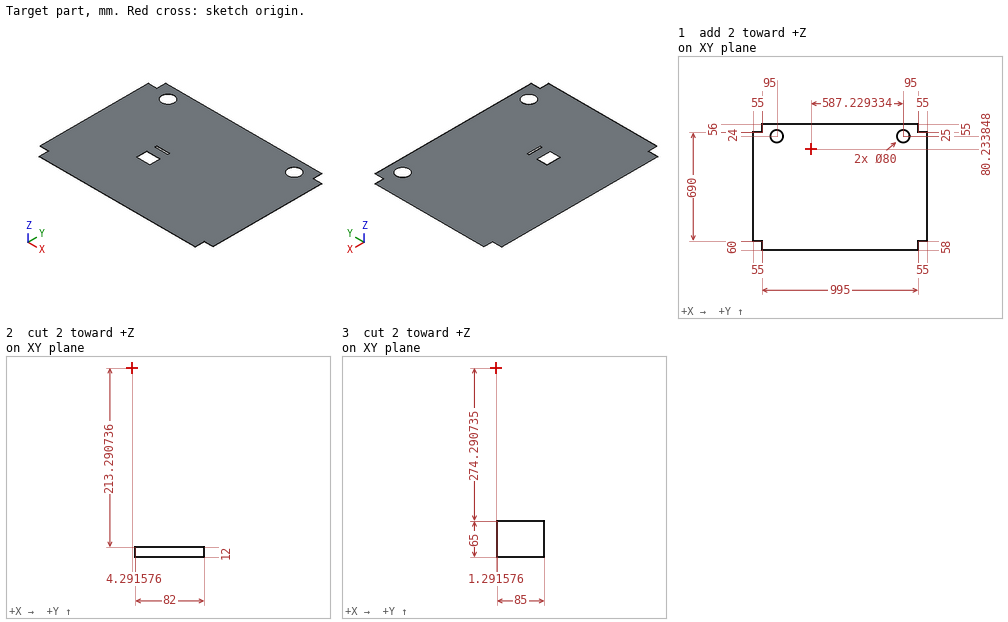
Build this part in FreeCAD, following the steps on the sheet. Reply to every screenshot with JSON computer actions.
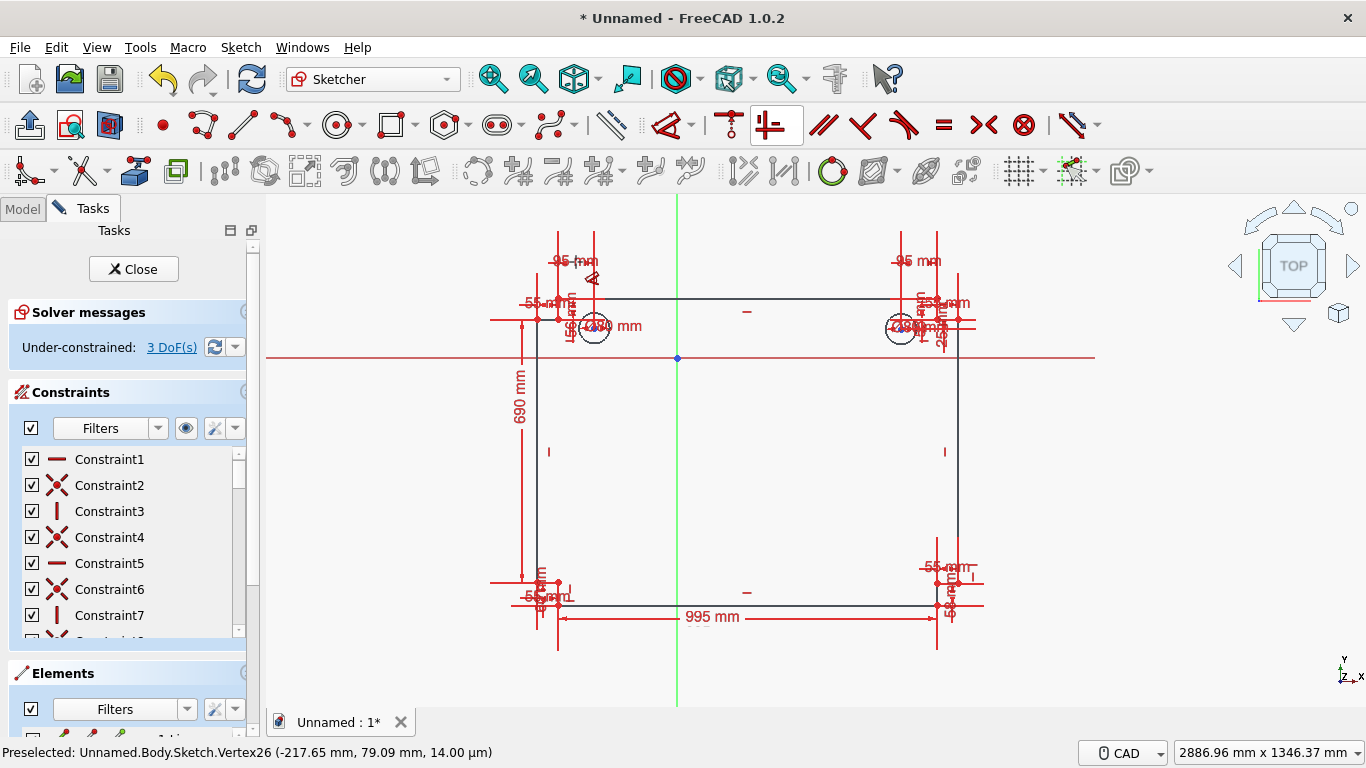
{"action": "scroll", "coordinate": [558, 320], "scroll_direction": "up", "scroll_amount": 8}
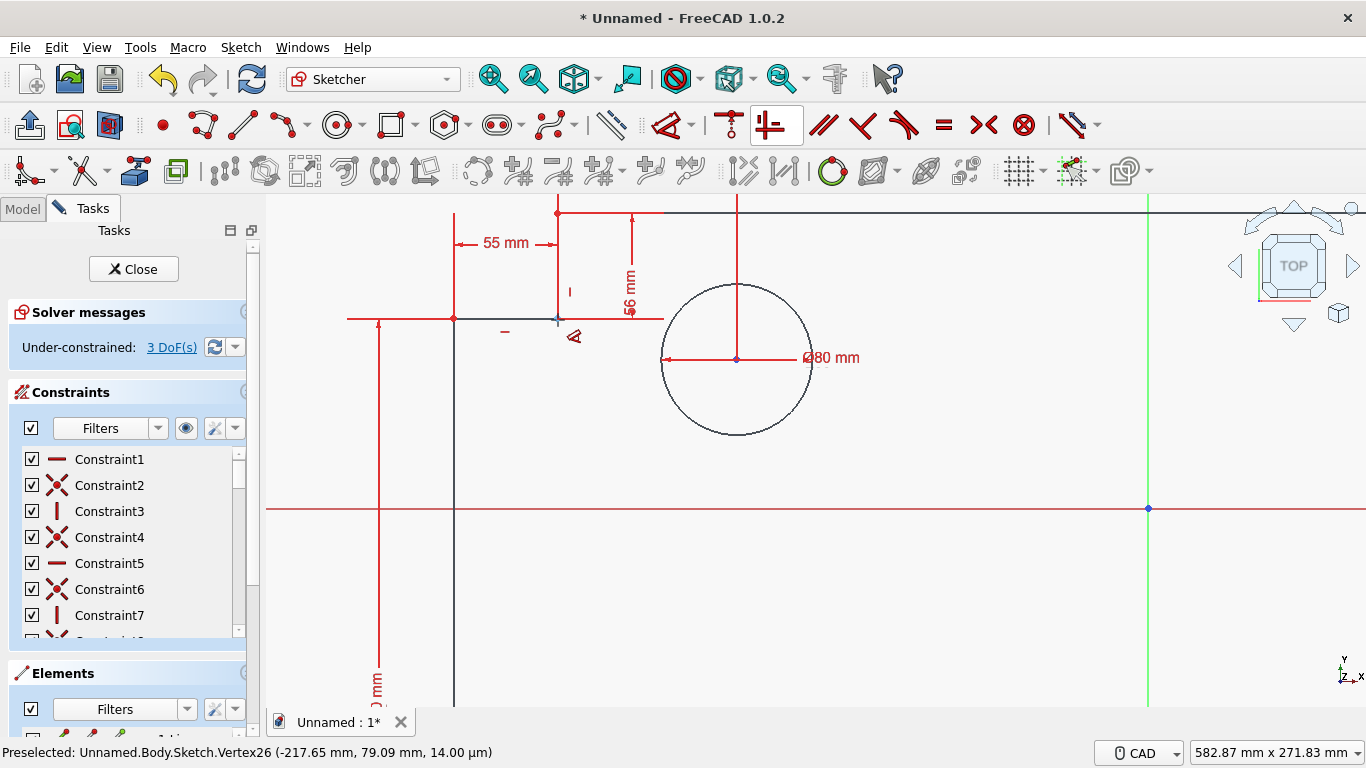
{"action": "left_click", "coordinate": [558, 319]}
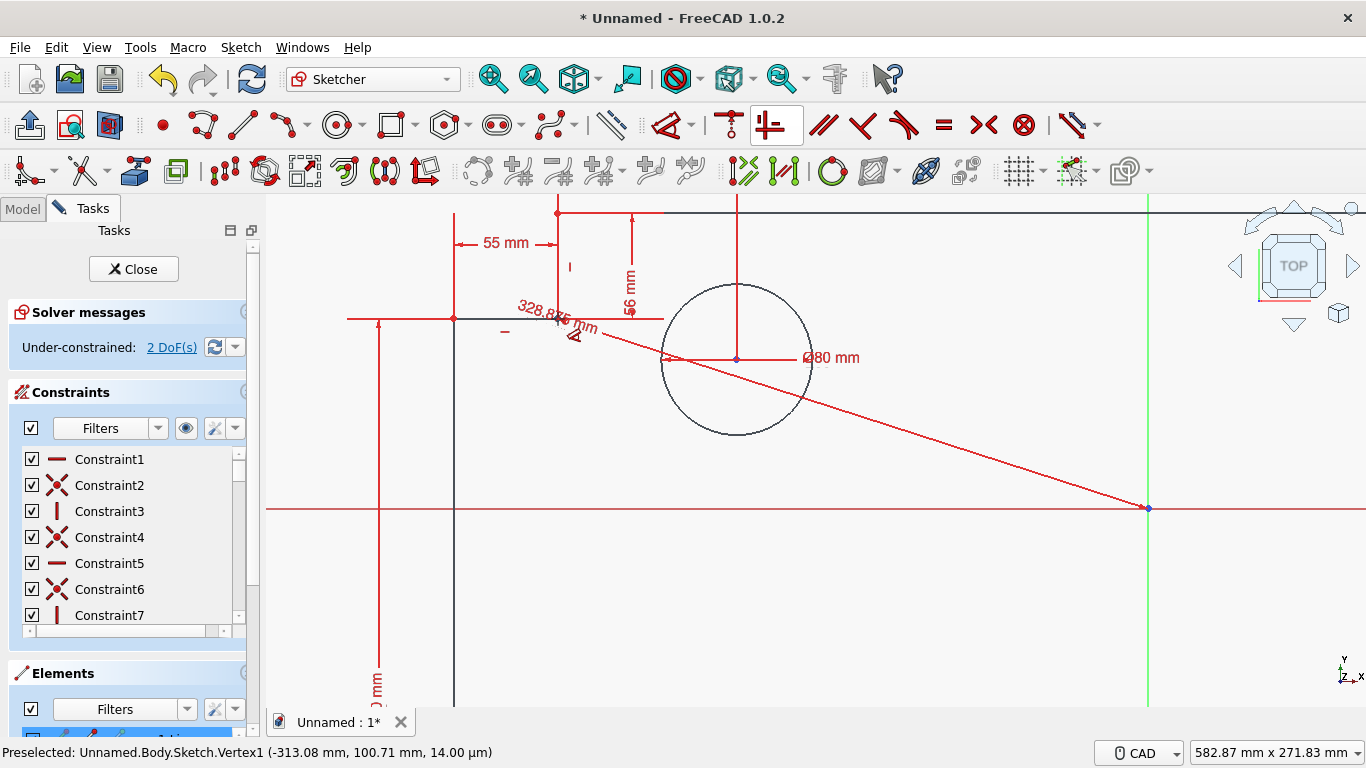
{"action": "left_click", "coordinate": [737, 360]}
{"action": "left_click", "coordinate": [524, 339]}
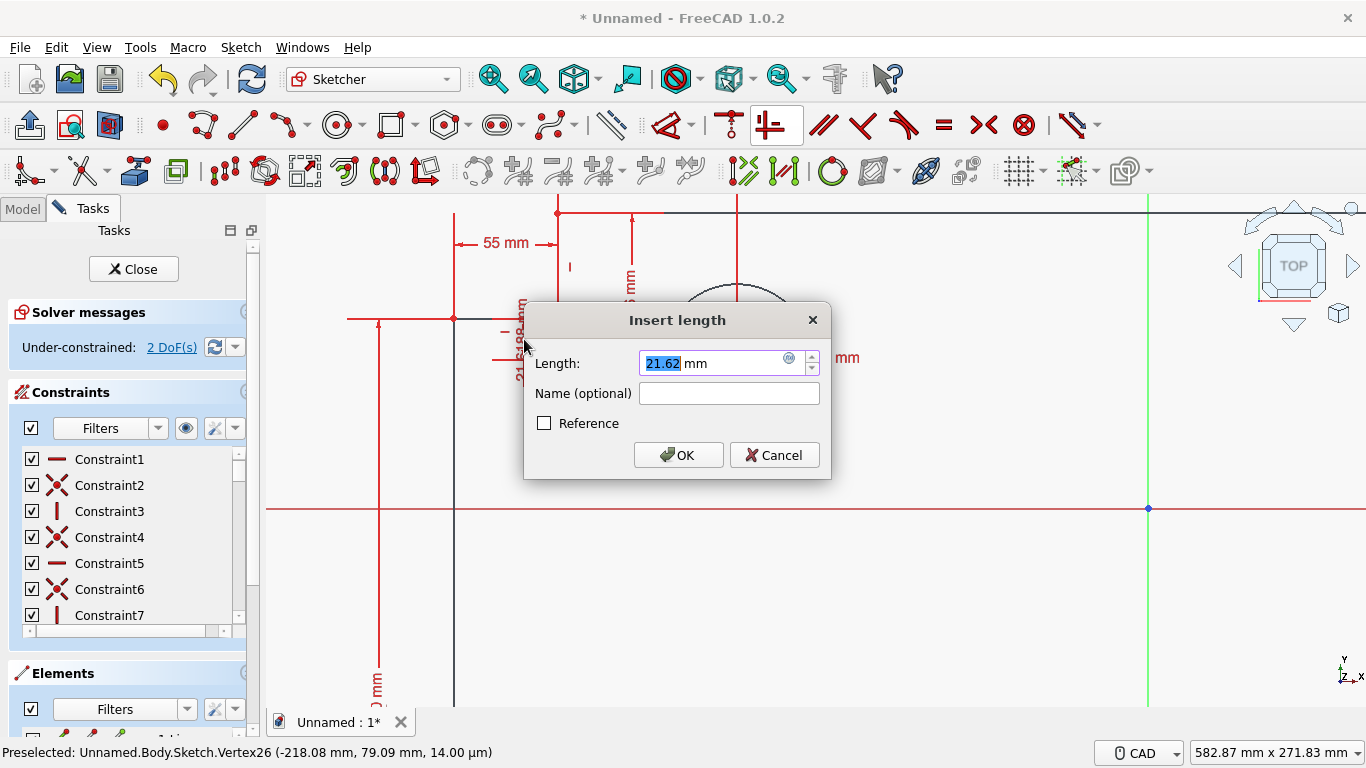
{"action": "type", "text": "24"}
{"action": "key", "text": "Return"}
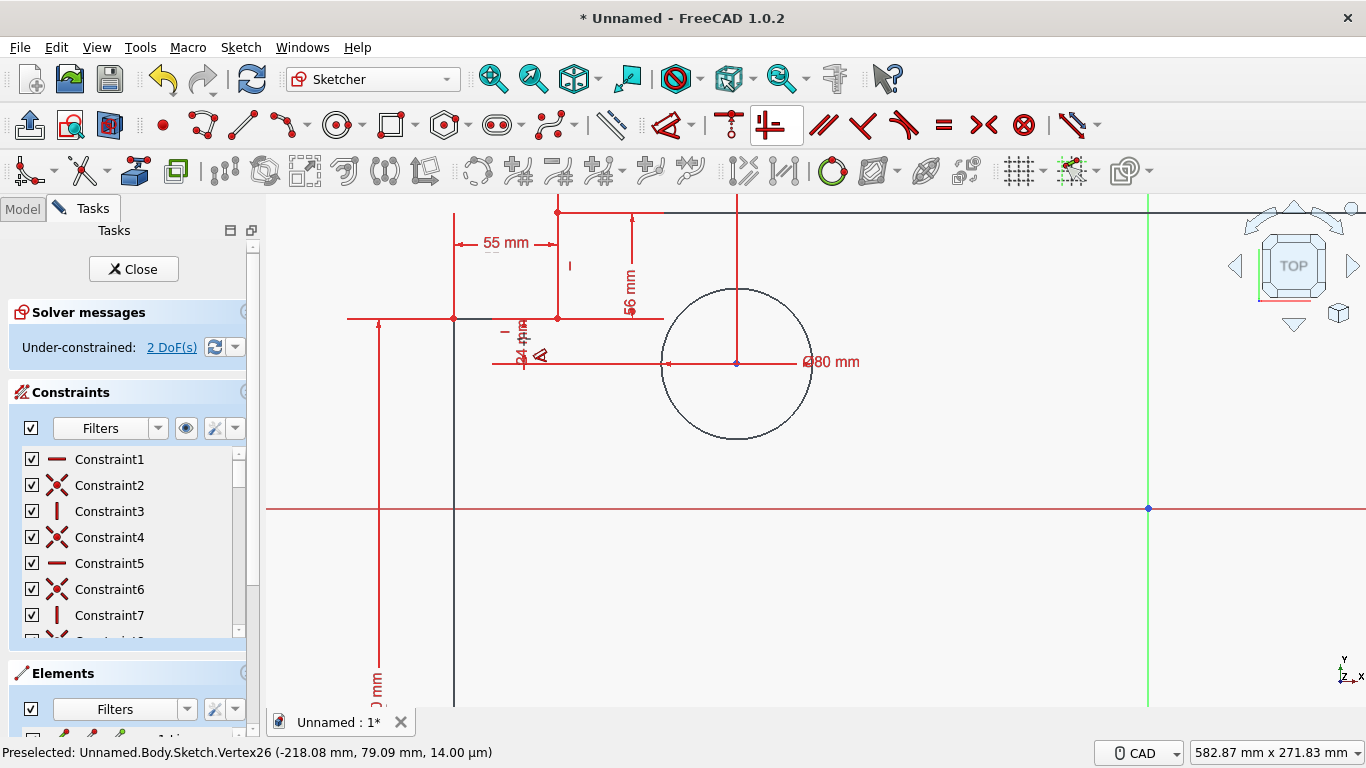
{"action": "scroll", "coordinate": [558, 320], "scroll_direction": "down", "scroll_amount": 8}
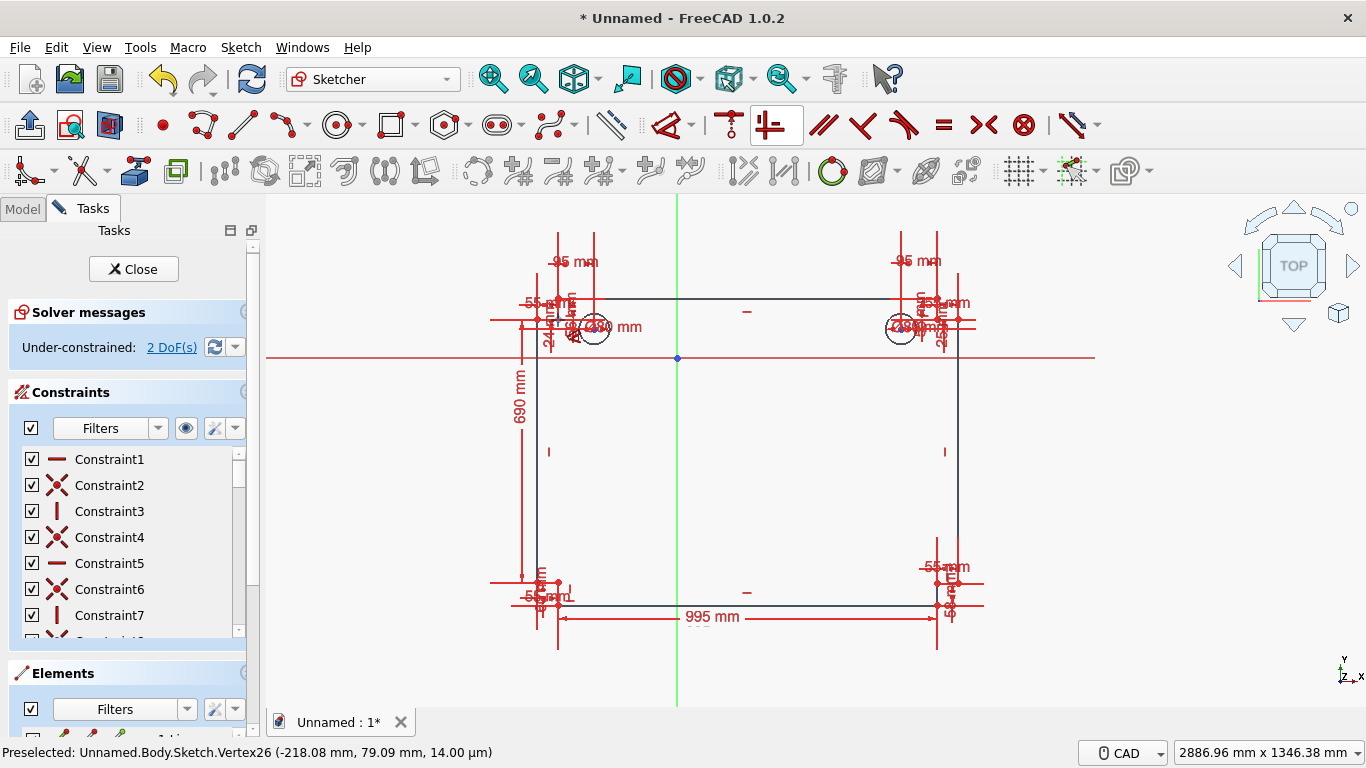
{"action": "scroll", "coordinate": [901, 329], "scroll_direction": "up", "scroll_amount": 2}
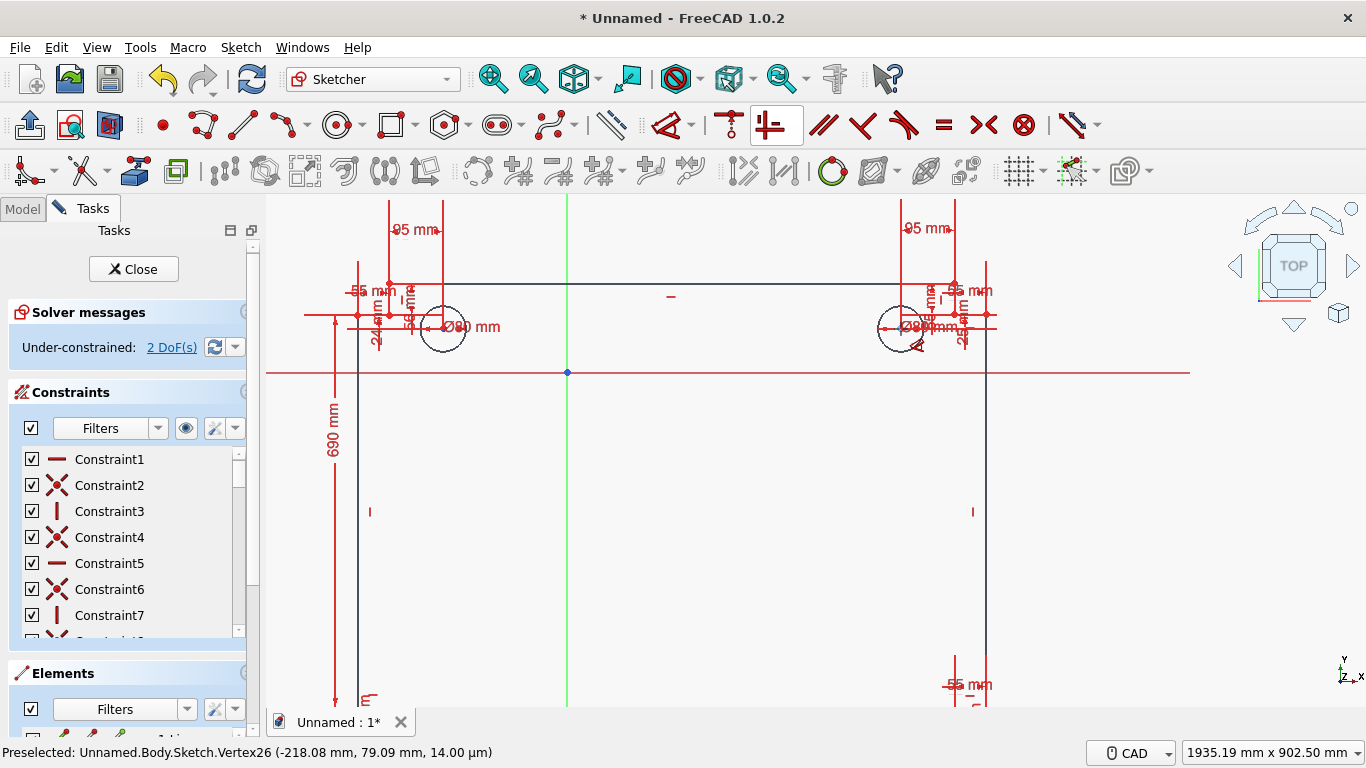
{"action": "left_click", "coordinate": [901, 329]}
{"action": "left_click", "coordinate": [935, 351]}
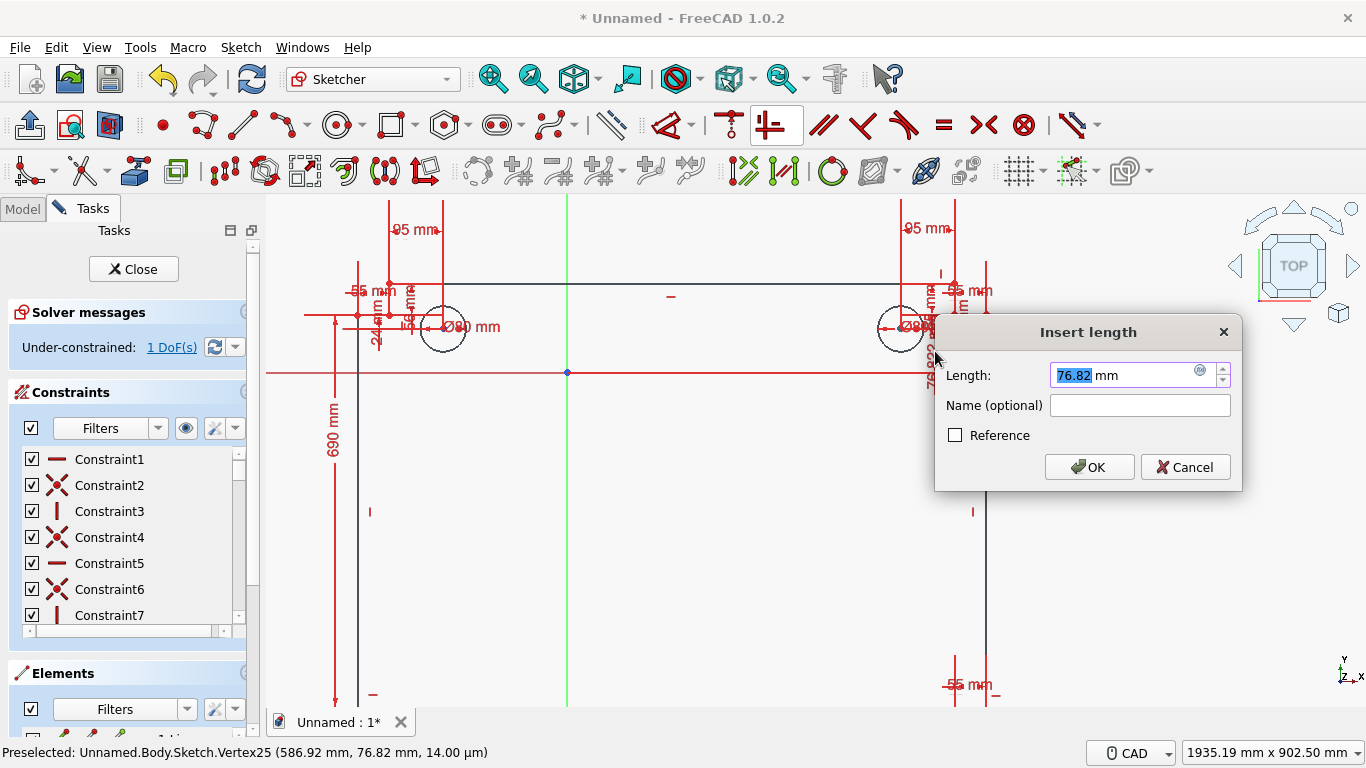
{"action": "type", "text": "80.233848"}
{"action": "key", "text": "Return"}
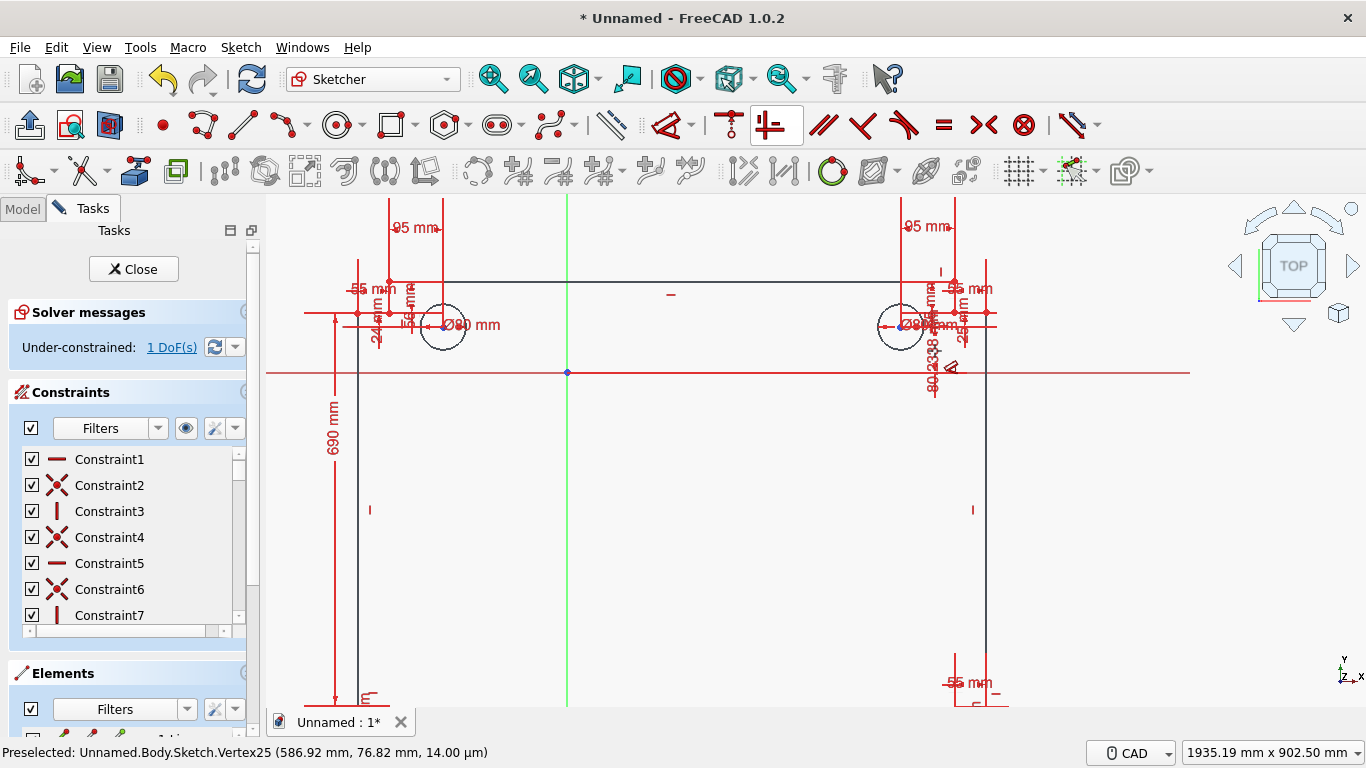
{"action": "left_click", "coordinate": [901, 327]}
{"action": "left_click", "coordinate": [734, 407]}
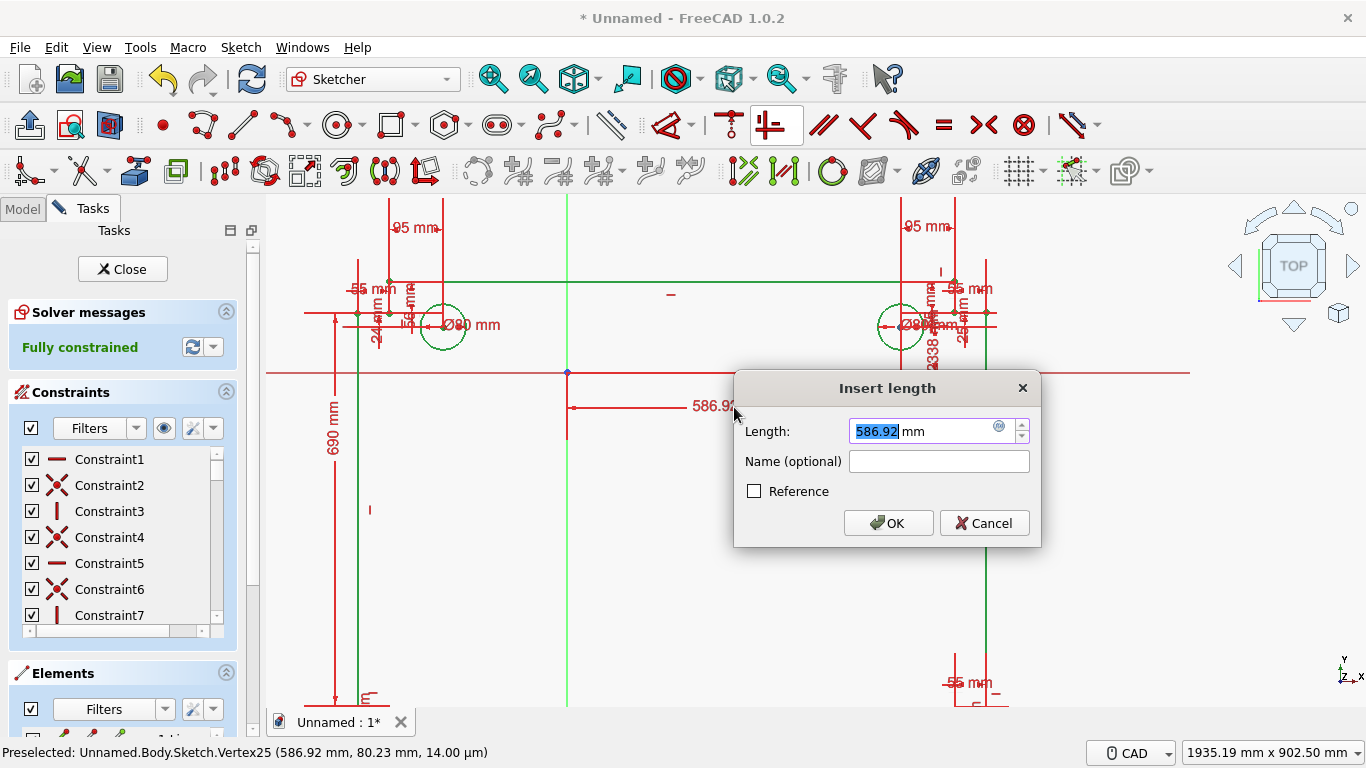
{"action": "type", "text": "587.229334"}
{"action": "key", "text": "Return"}
{"action": "key", "text": "Escape"}